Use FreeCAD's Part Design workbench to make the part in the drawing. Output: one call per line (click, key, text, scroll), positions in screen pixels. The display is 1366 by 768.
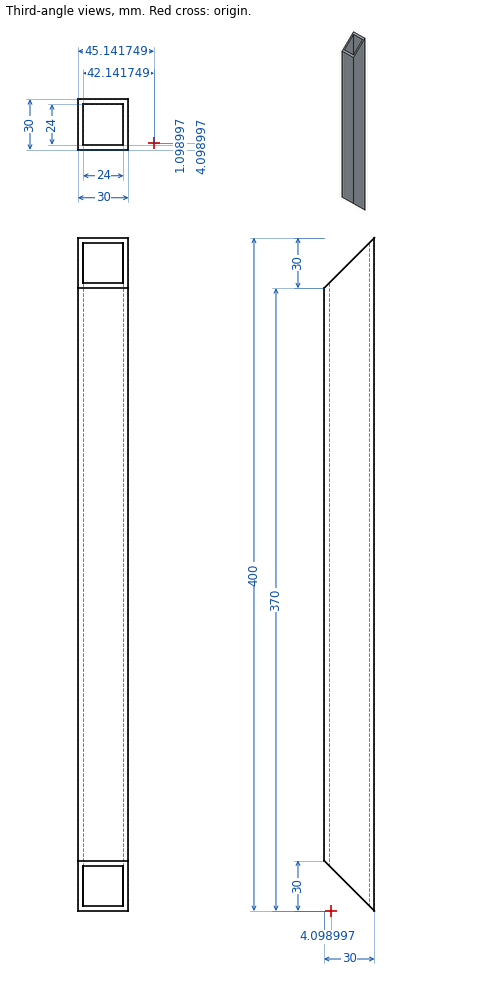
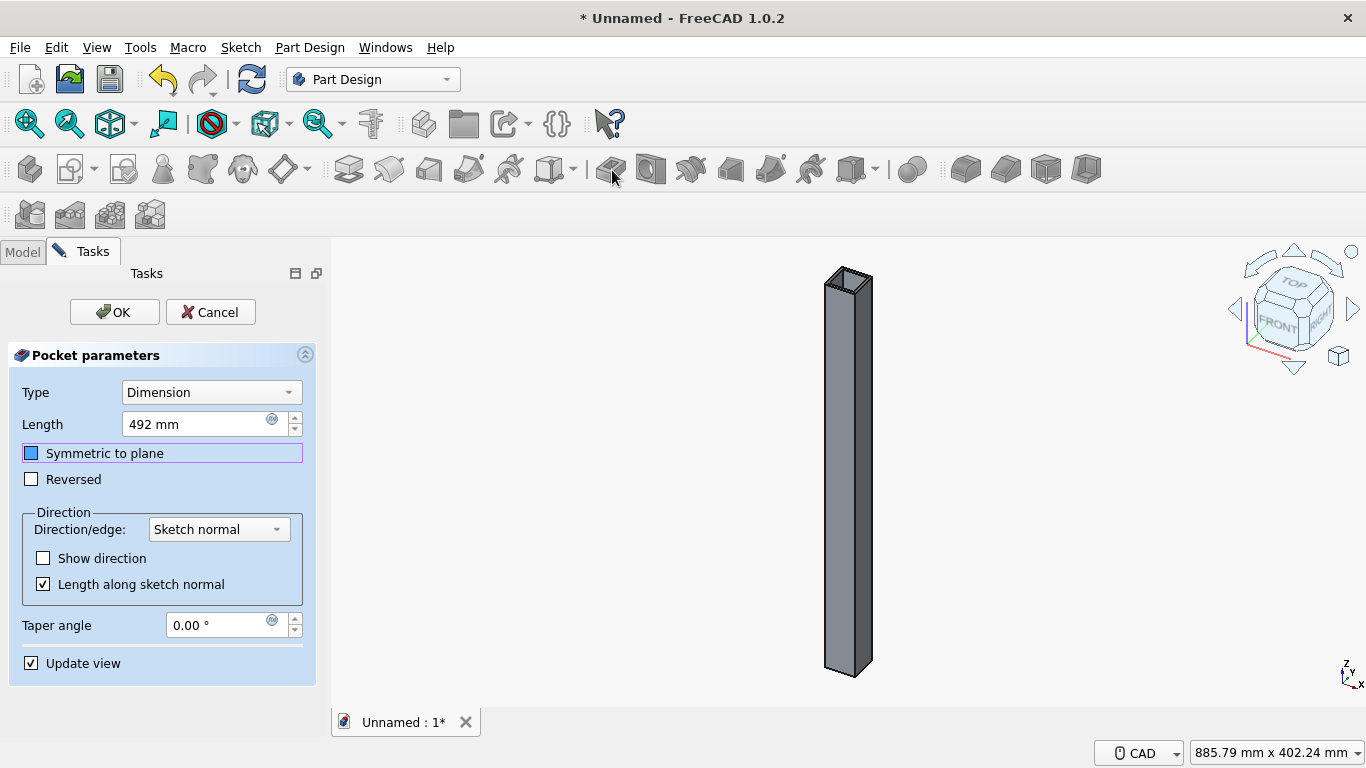
click(115, 312)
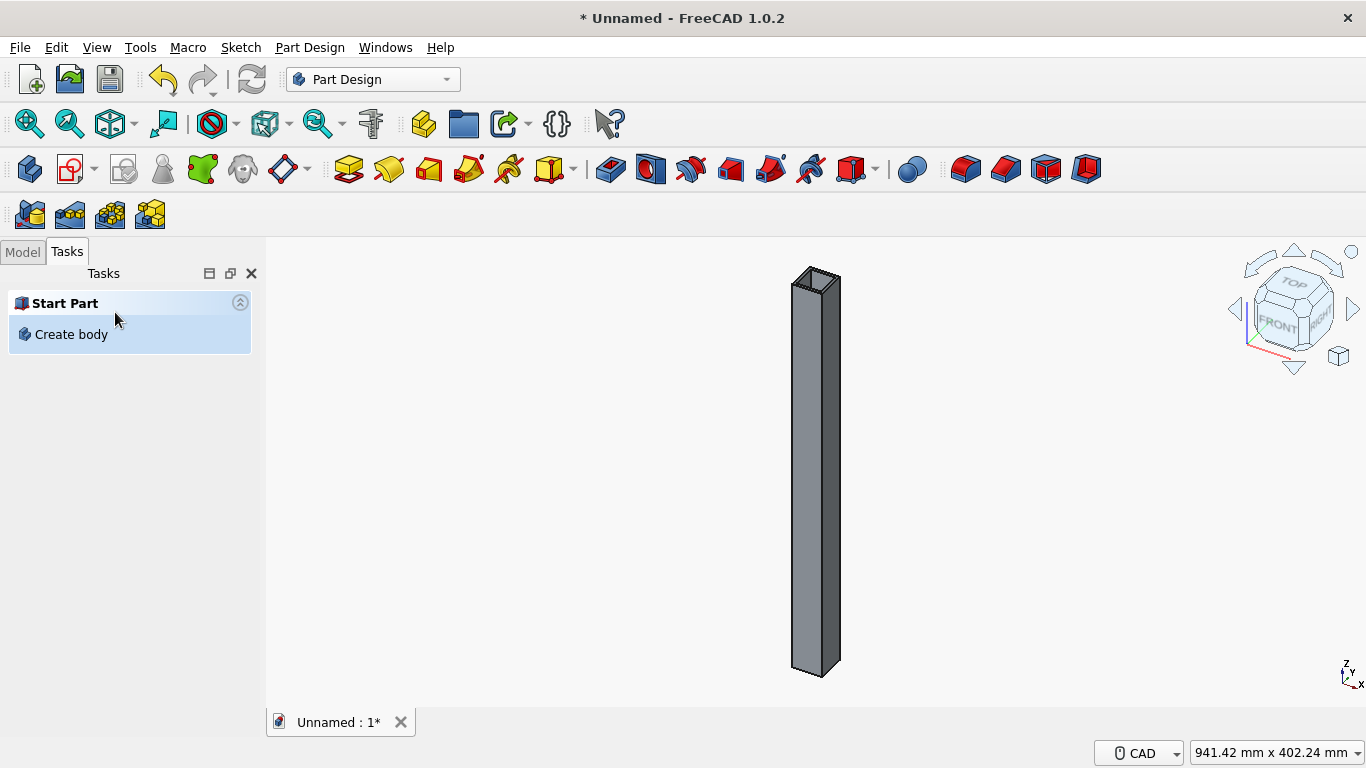
click(831, 312)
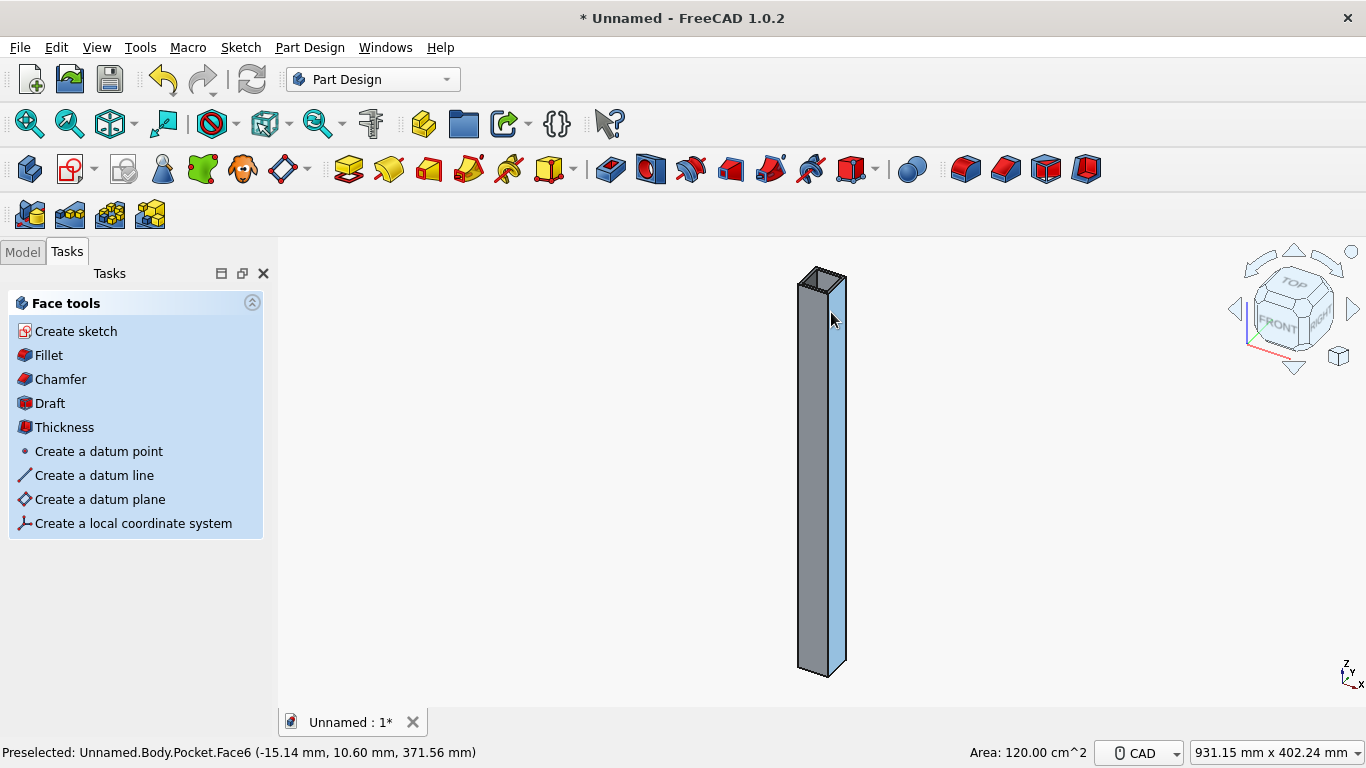
click(70, 170)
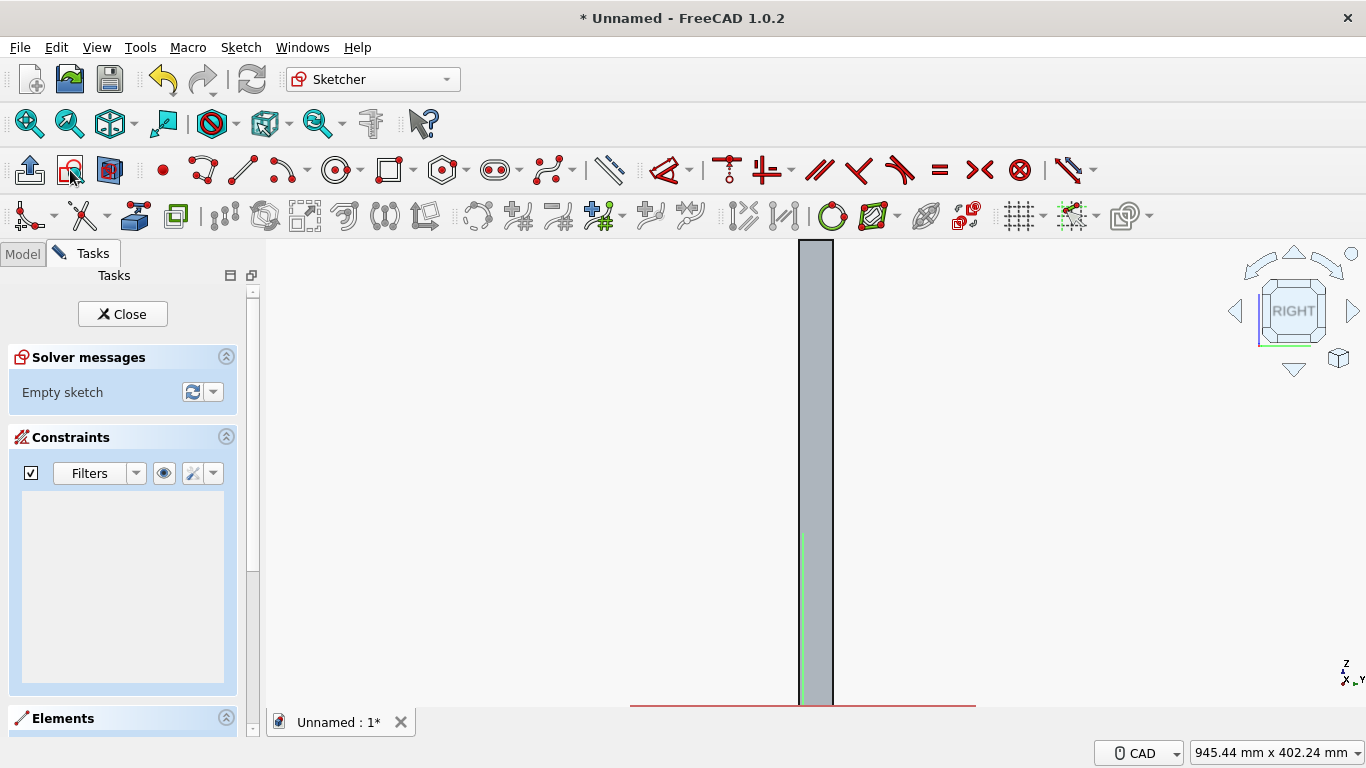
scroll(748, 473, down, 5)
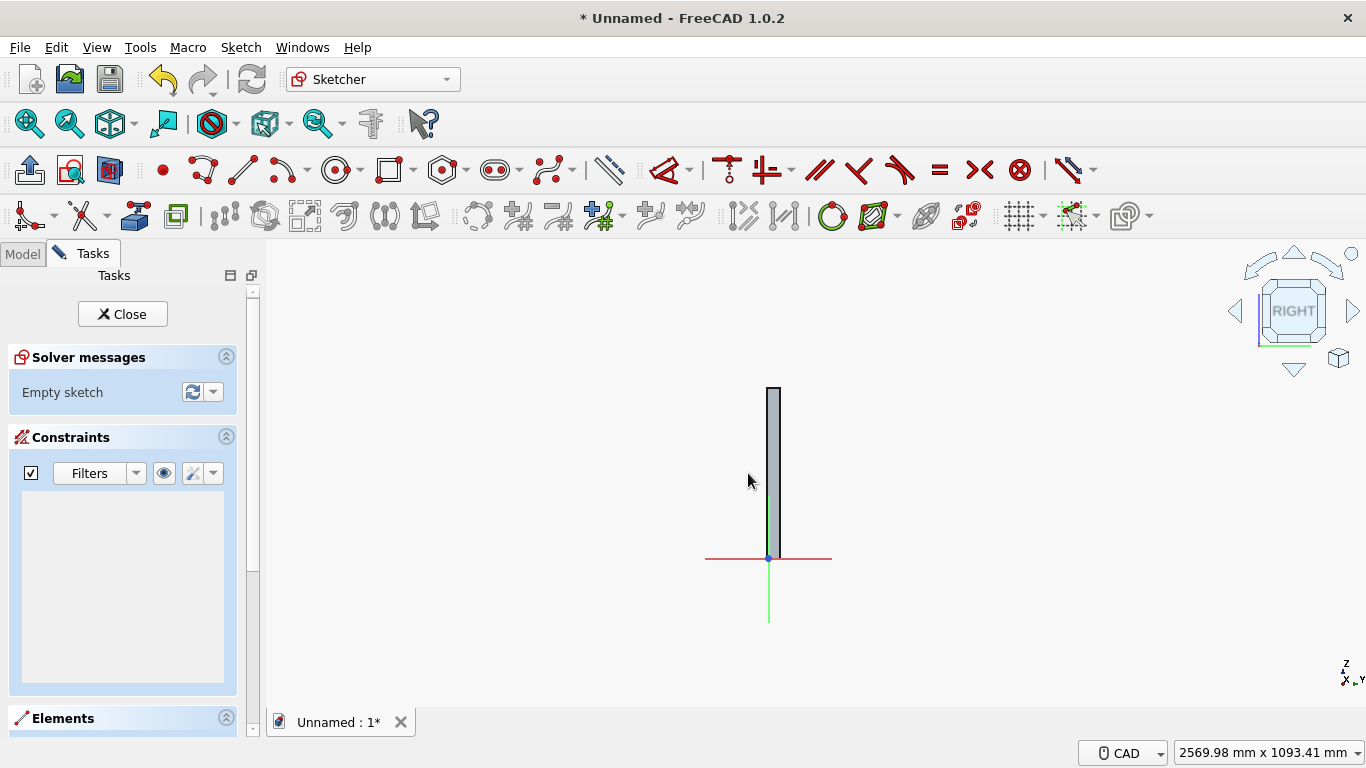
scroll(775, 557, up, 15)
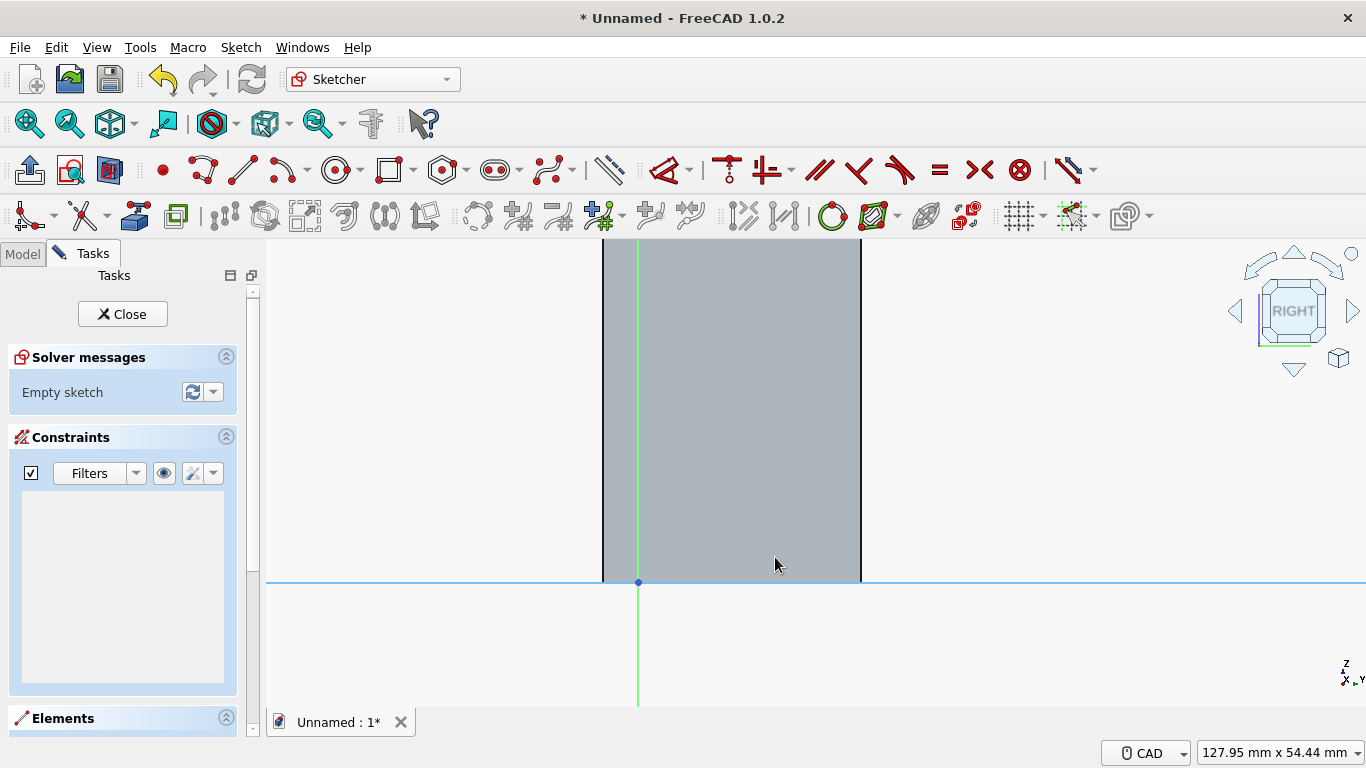
click(204, 170)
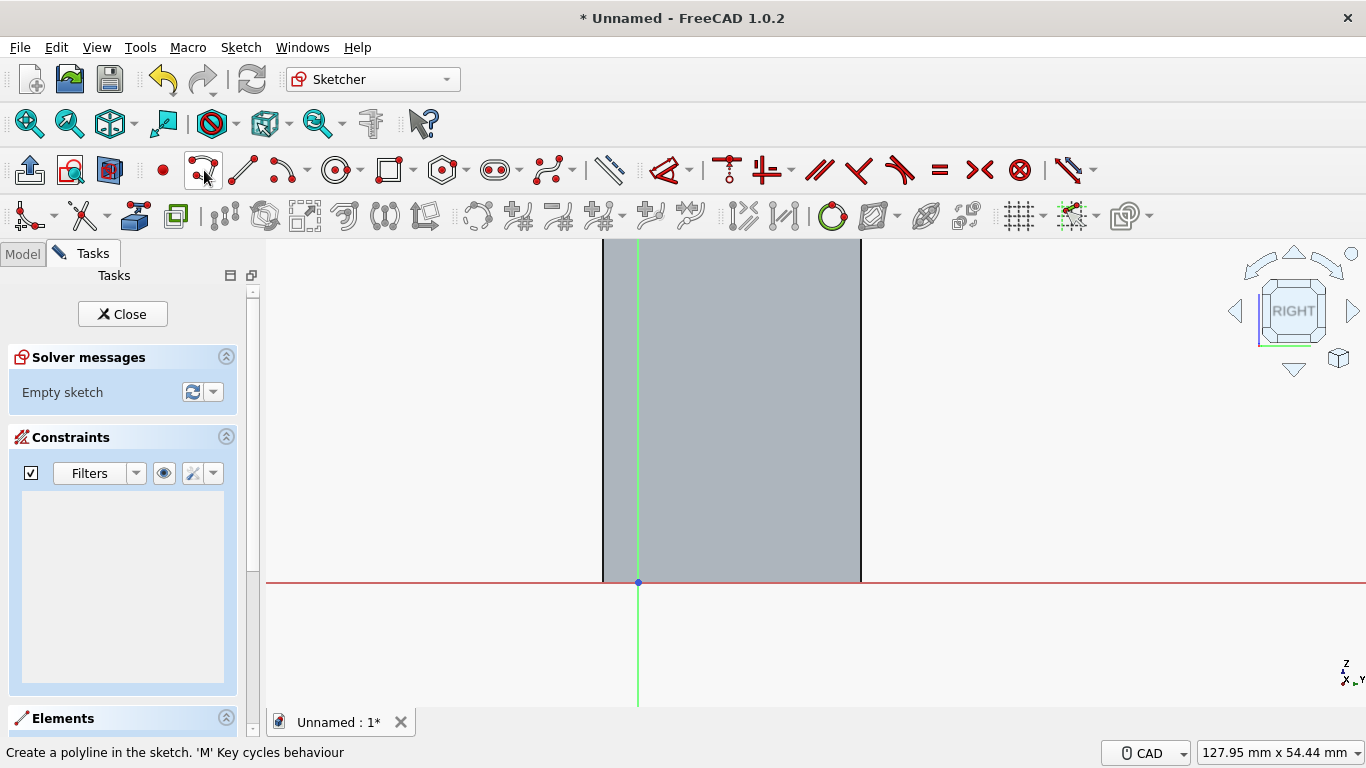
click(603, 583)
click(861, 574)
click(603, 325)
click(603, 583)
key(Escape)
key(Escape)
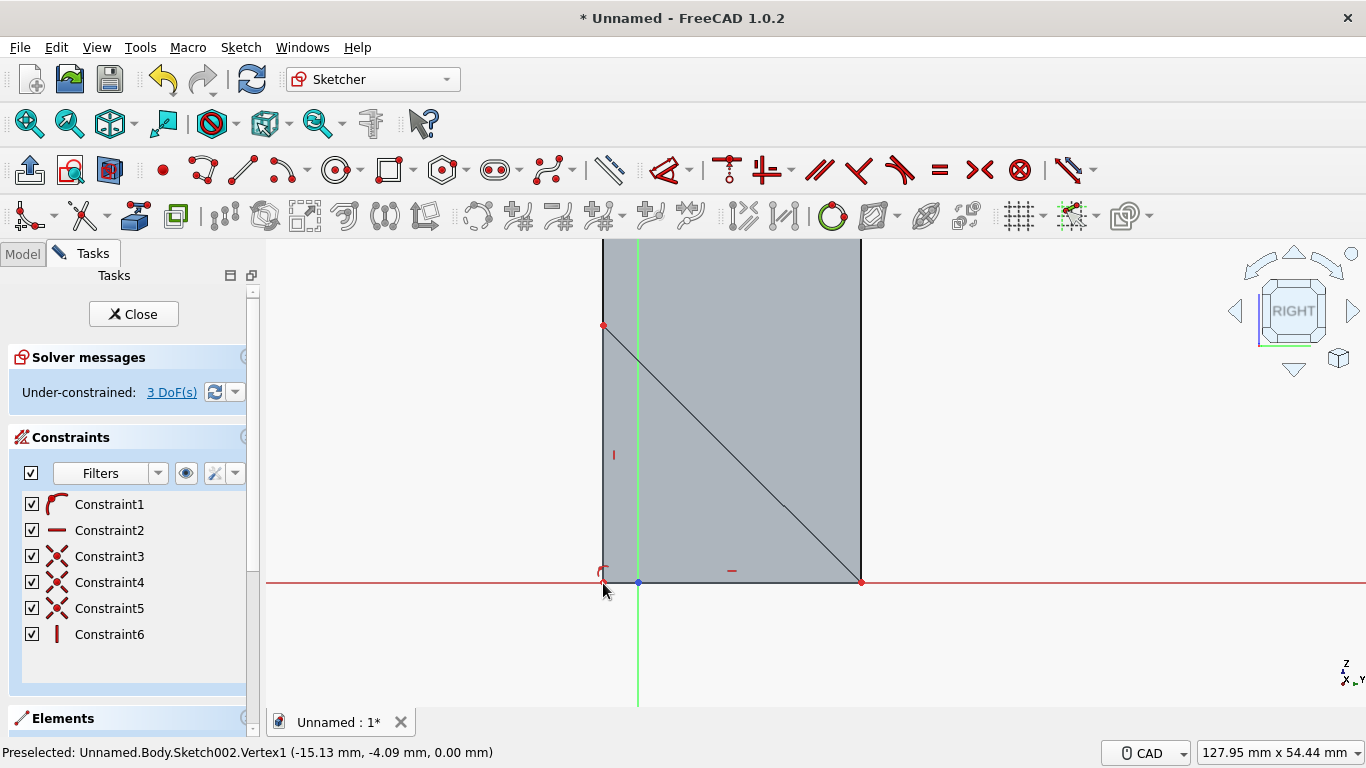
key(d)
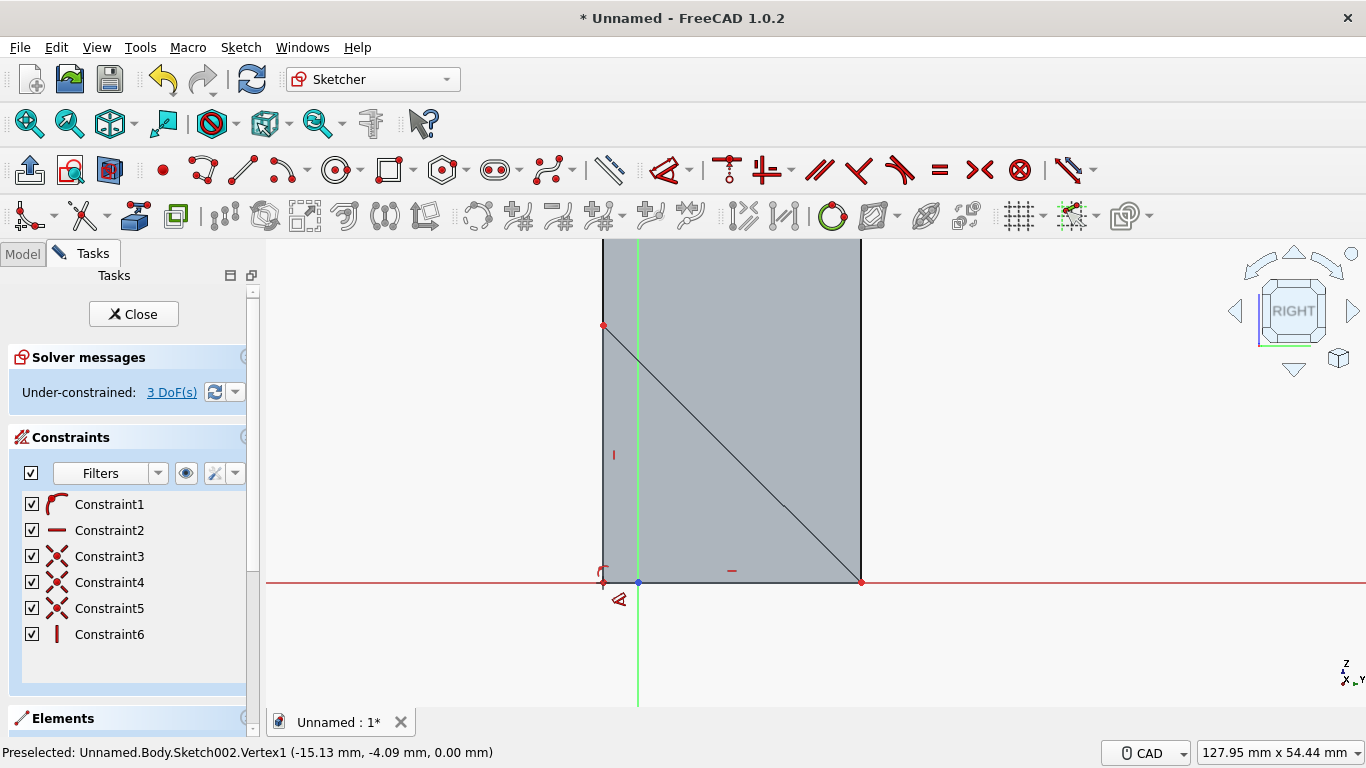
click(680, 583)
click(732, 617)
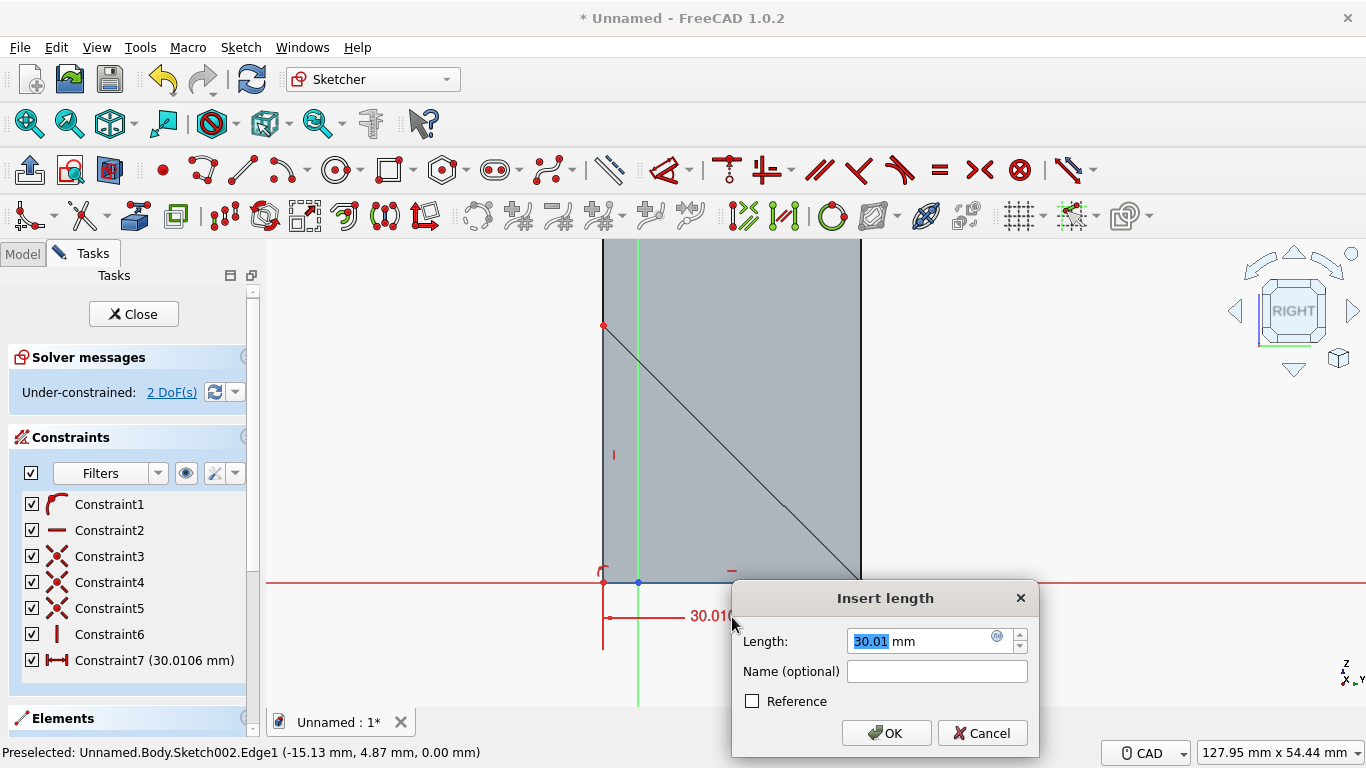
text(30)
key(Return)